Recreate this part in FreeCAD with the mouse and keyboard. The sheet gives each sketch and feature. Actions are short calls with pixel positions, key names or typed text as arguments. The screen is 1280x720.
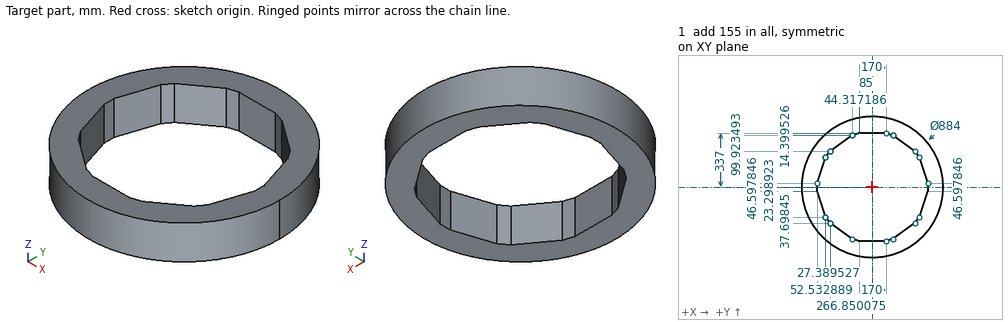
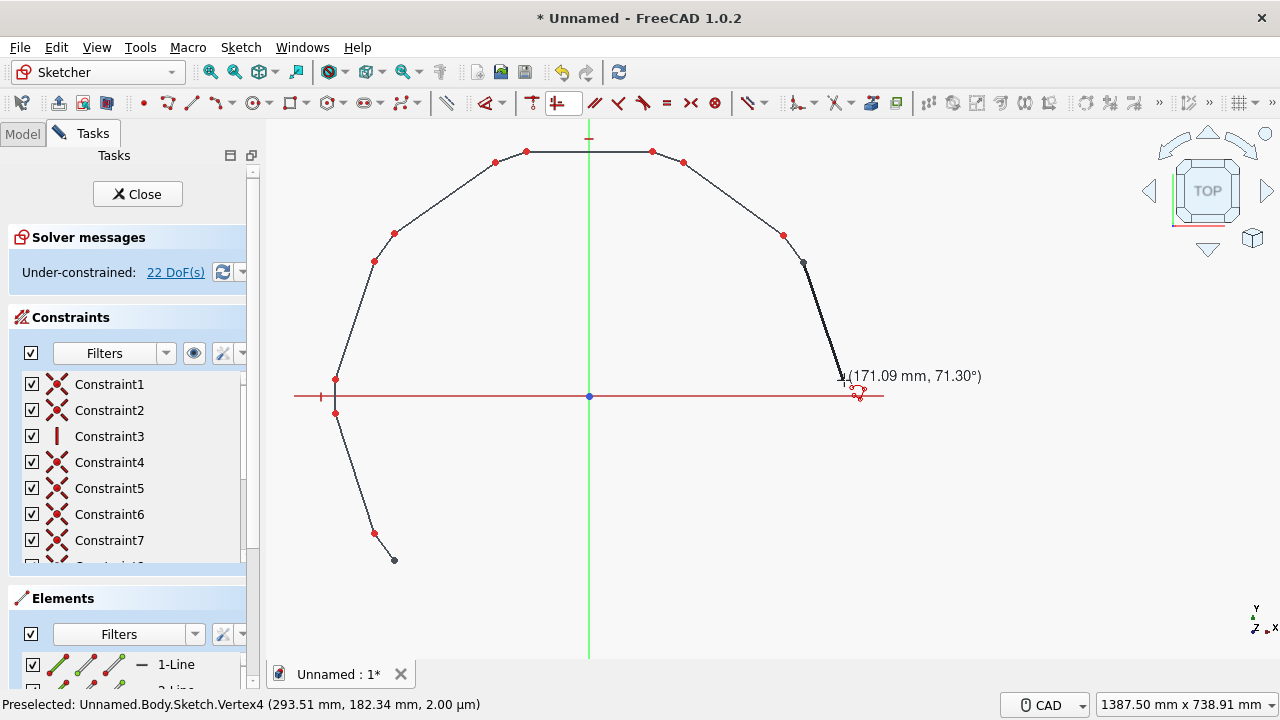
click(843, 379)
click(843, 413)
click(804, 531)
click(784, 559)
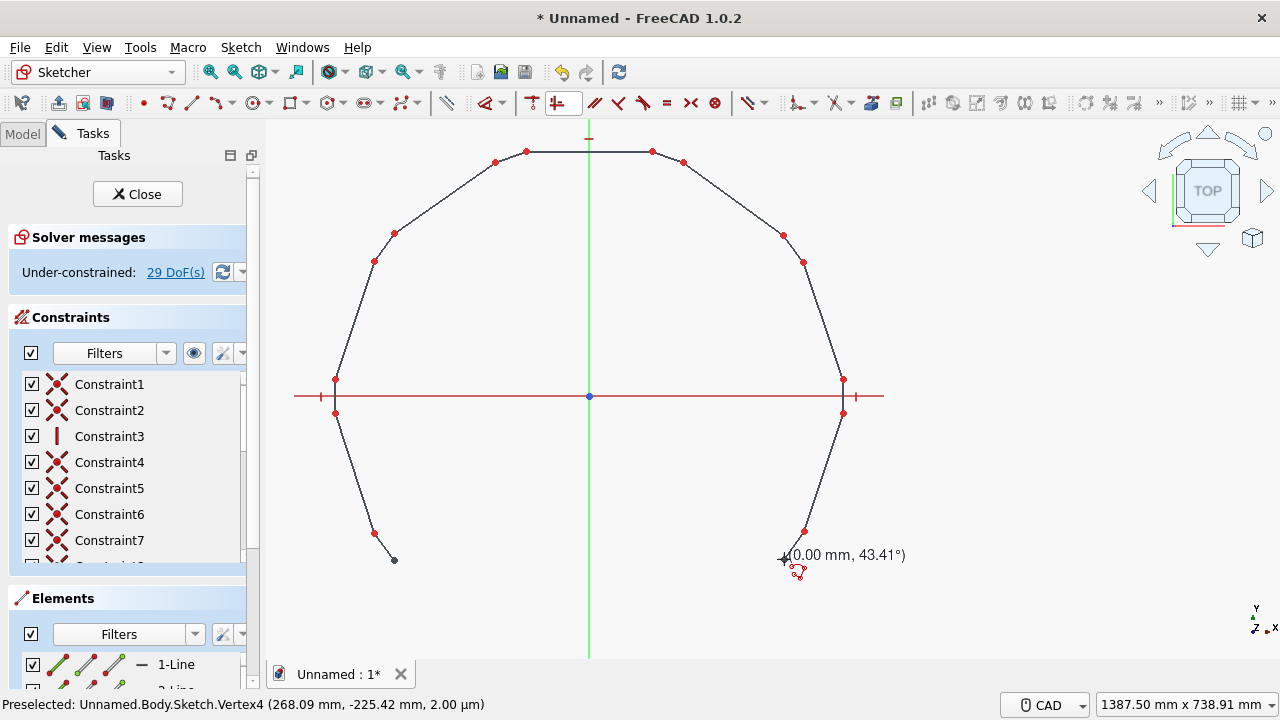
scroll(845, 380, down, 3)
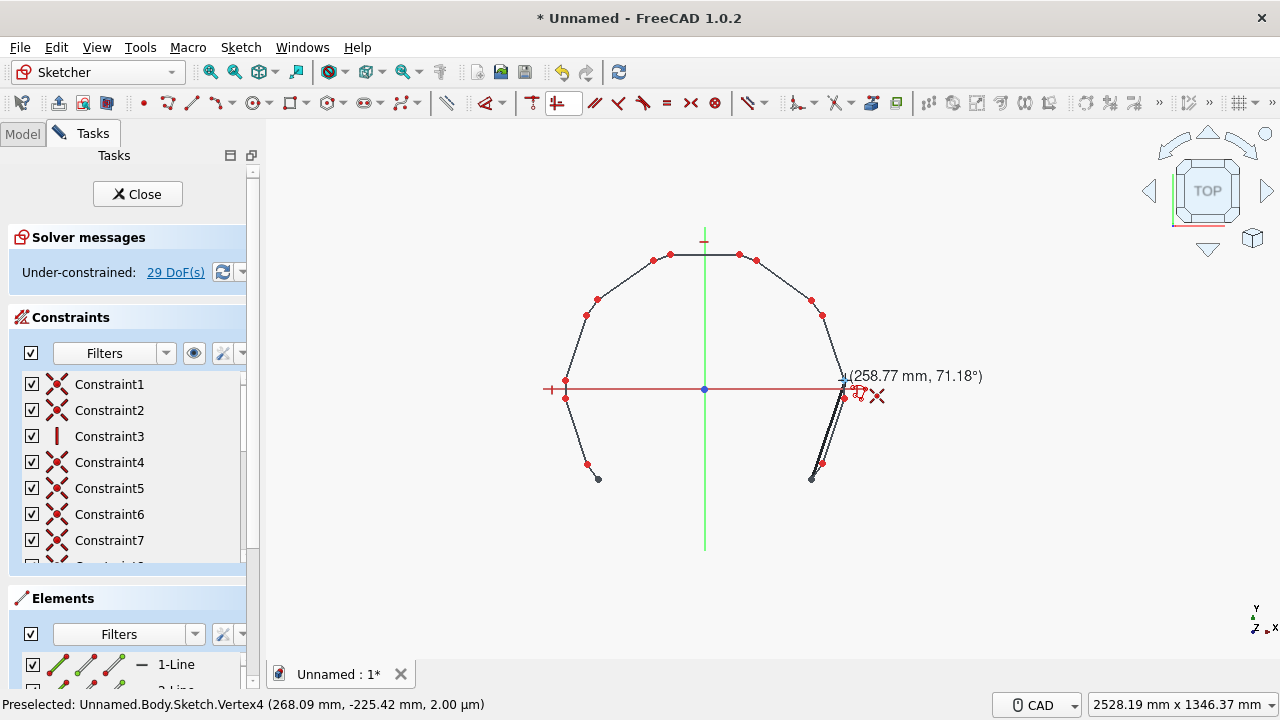
click(757, 518)
click(739, 524)
click(671, 524)
click(653, 518)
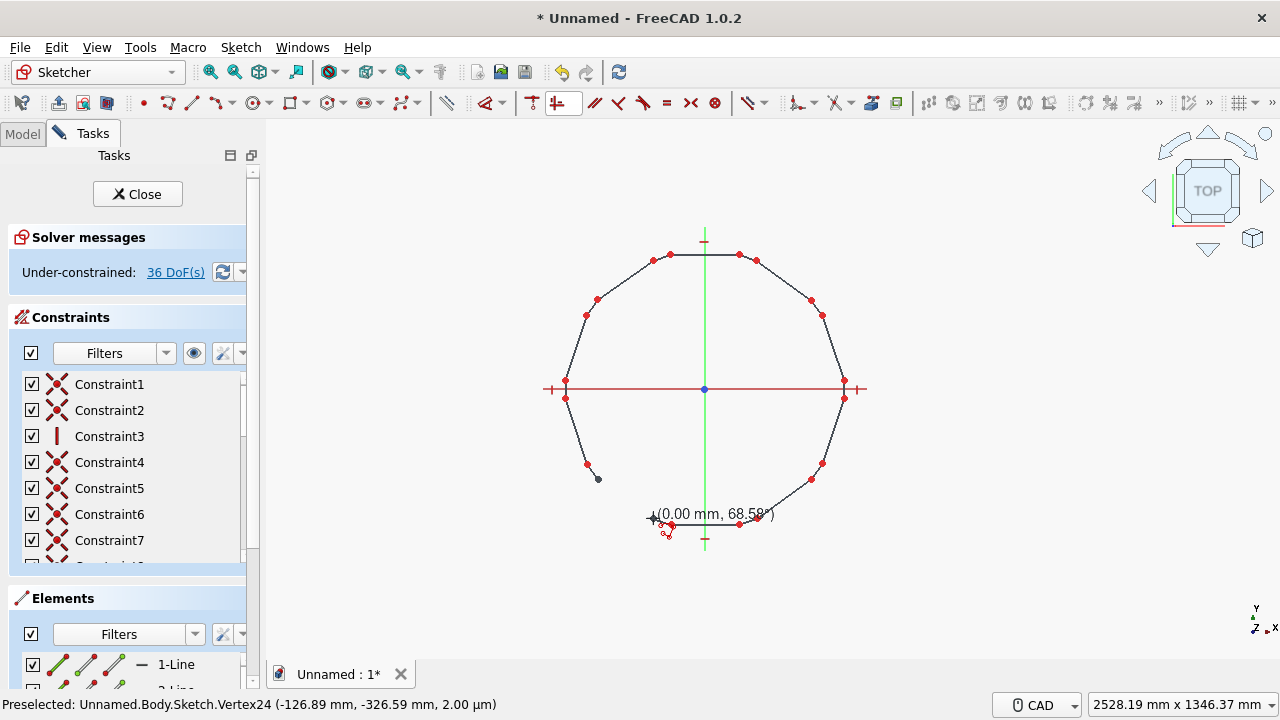
scroll(598, 478, up, 3)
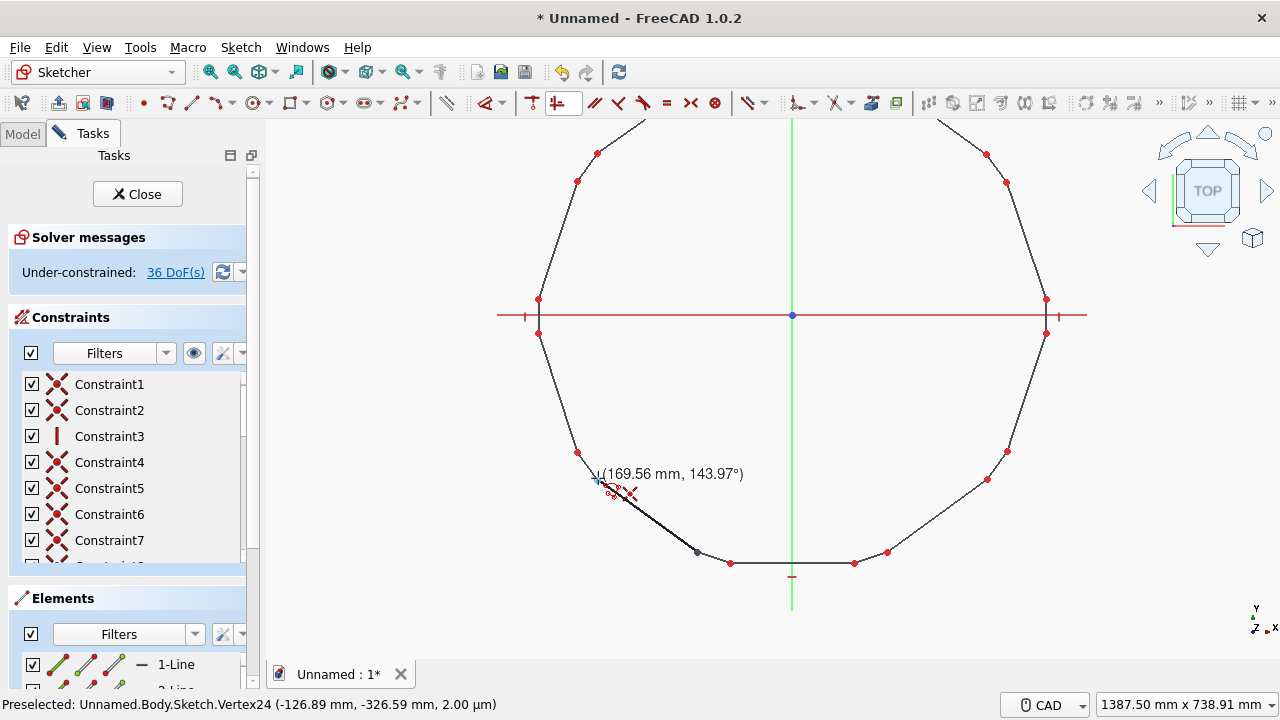
click(598, 480)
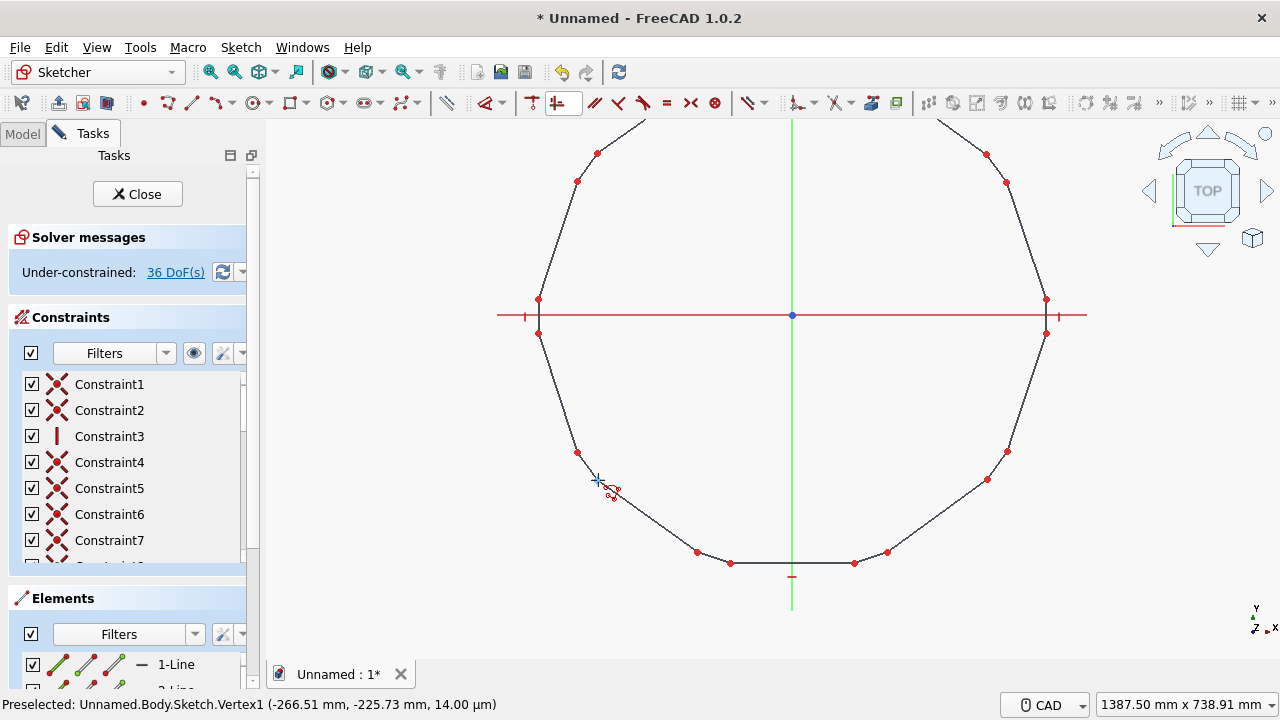
click(254, 104)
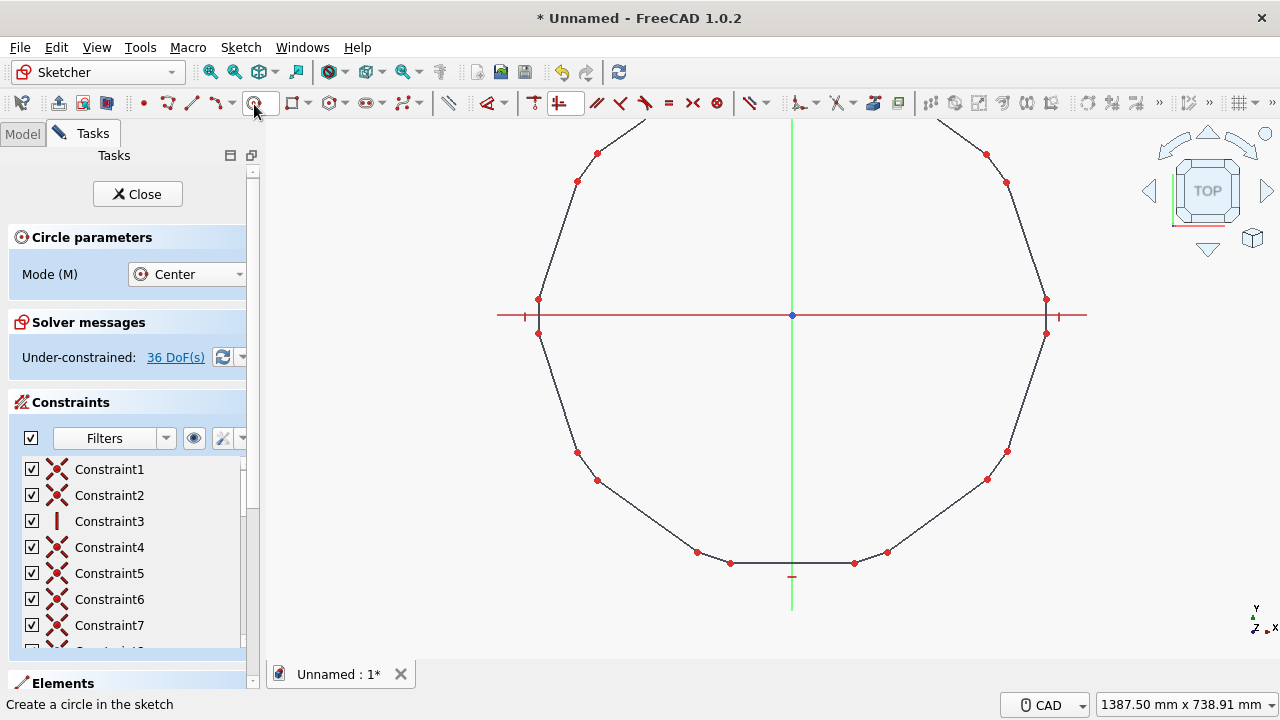
click(793, 315)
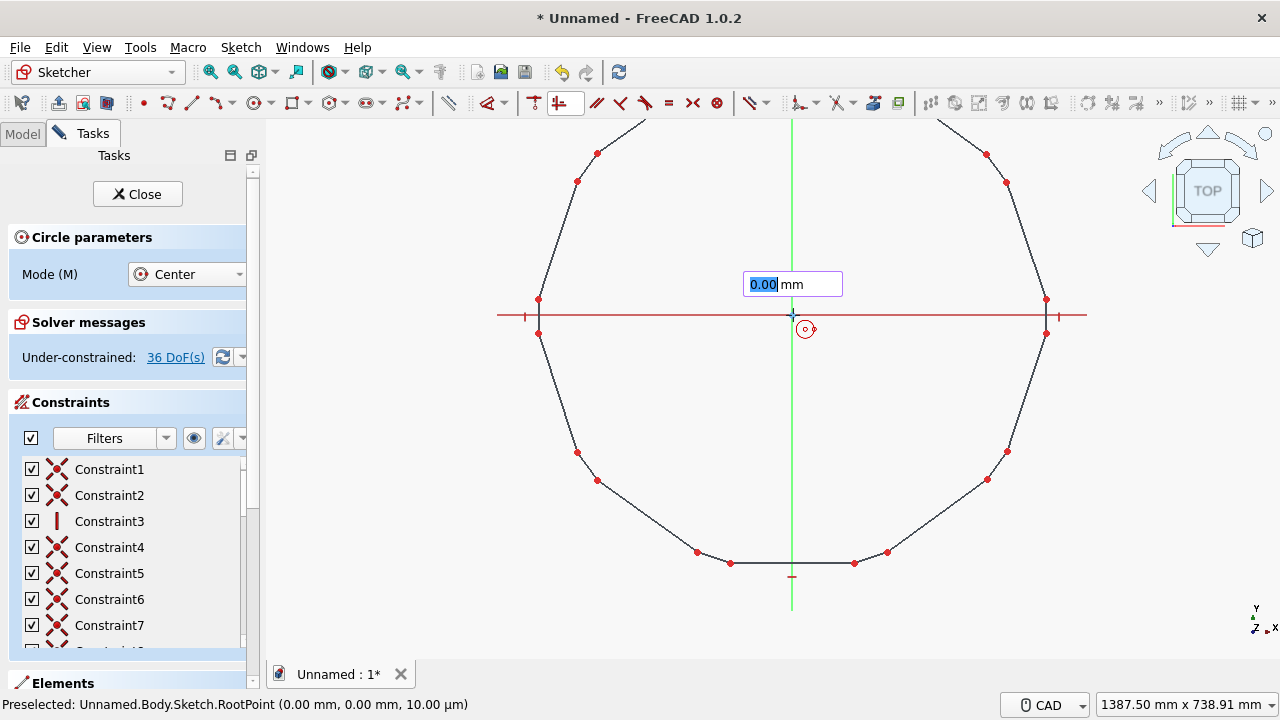
scroll(597, 479, down, 3)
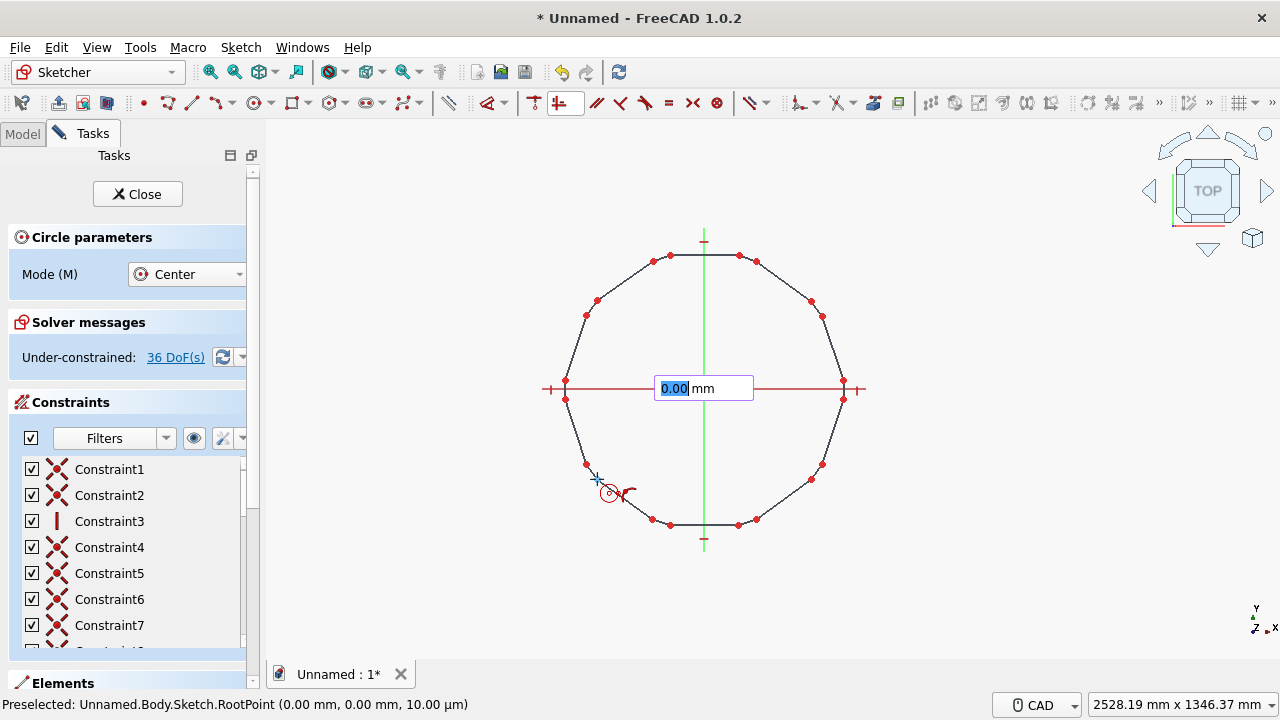
click(830, 264)
key(Escape)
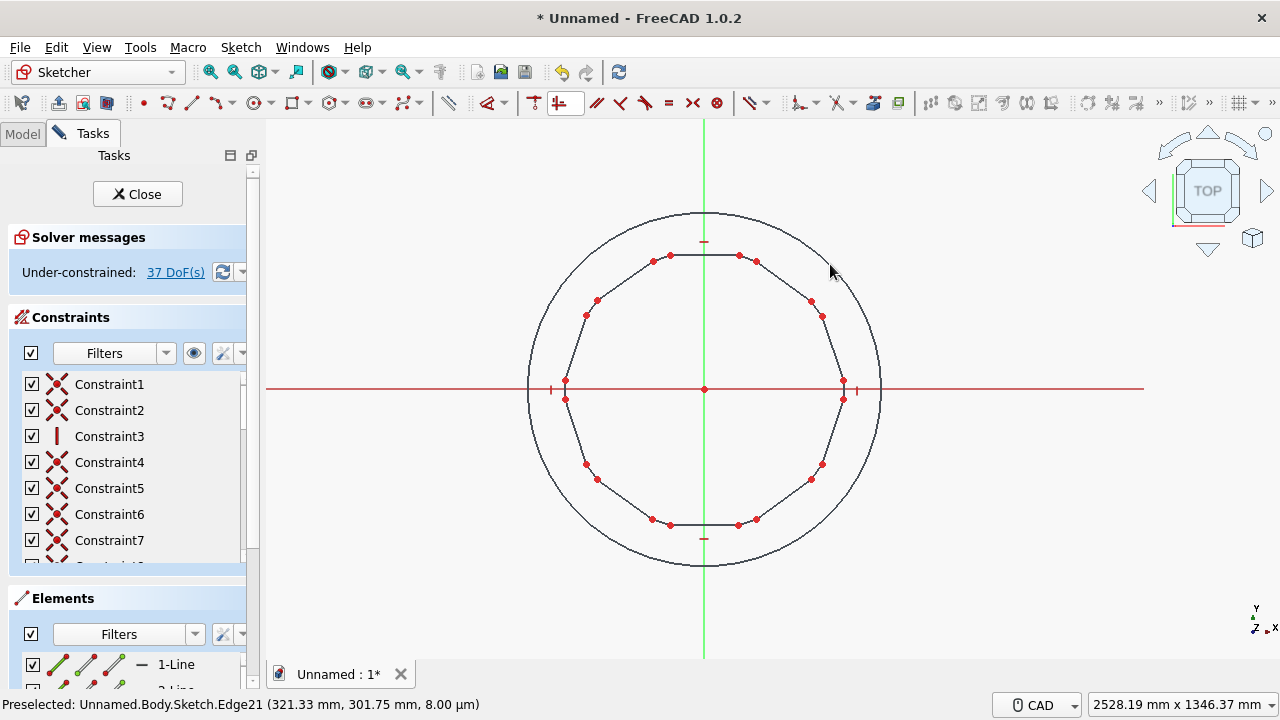
click(587, 465)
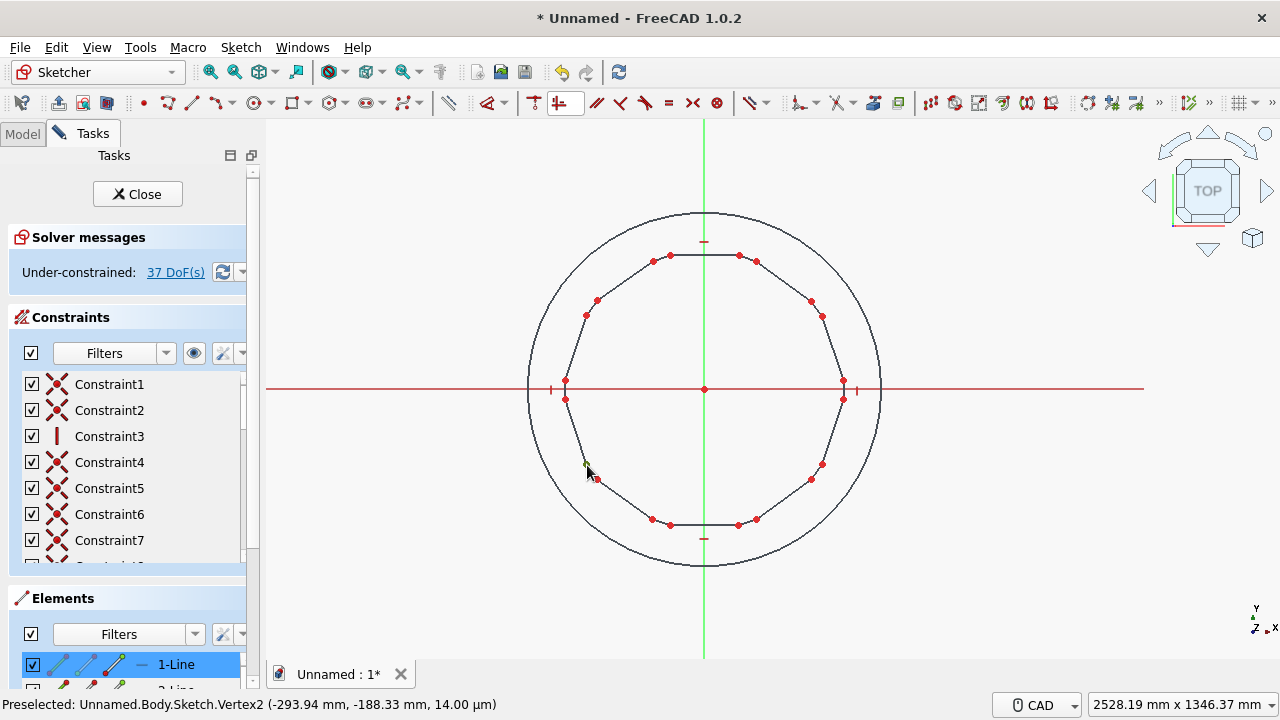
click(587, 316)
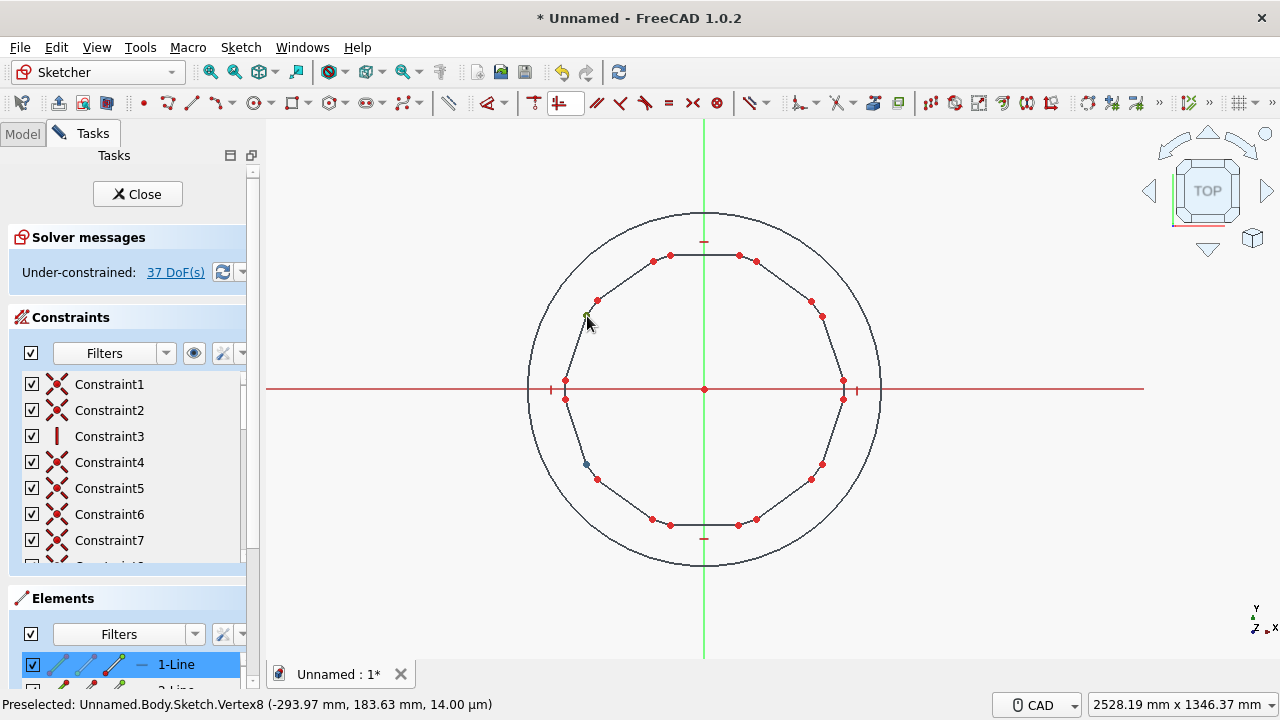
click(353, 389)